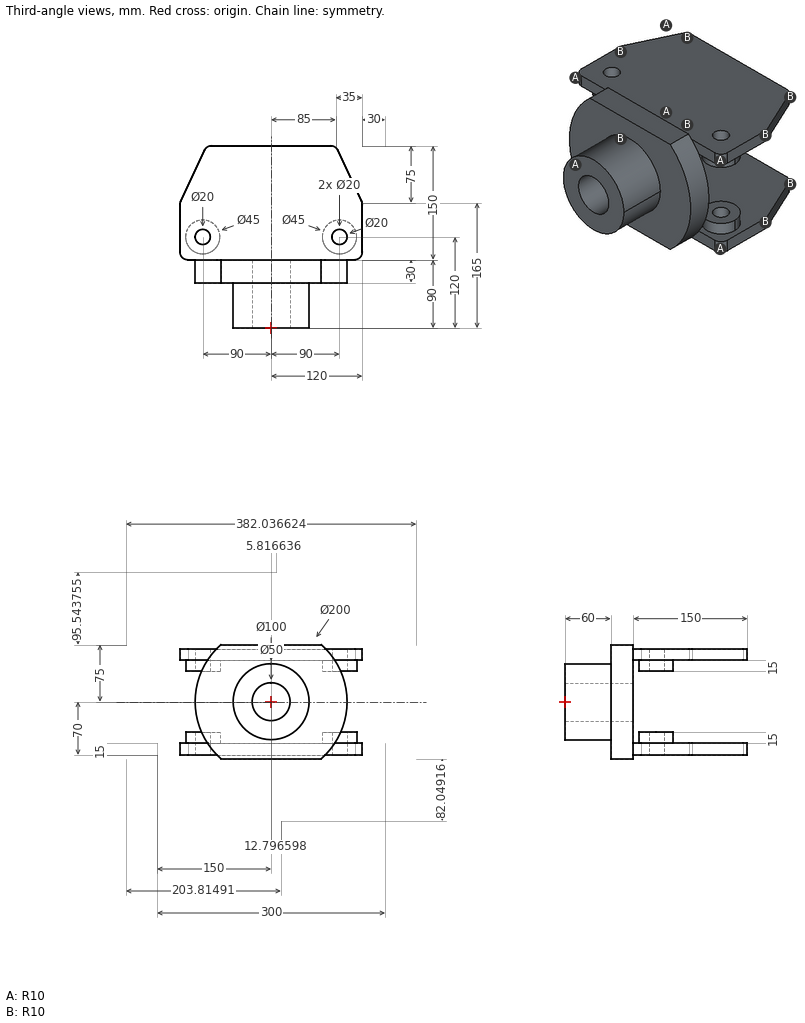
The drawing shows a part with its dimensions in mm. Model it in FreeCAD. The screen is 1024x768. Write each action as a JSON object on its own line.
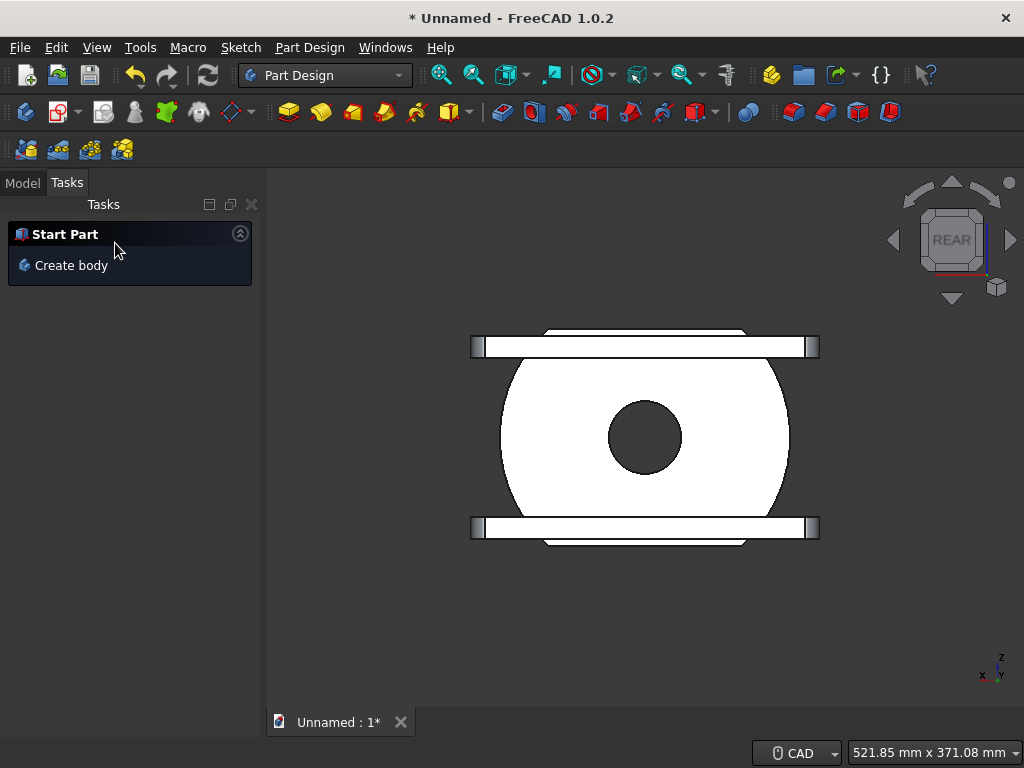
{"action": "key", "text": "5"}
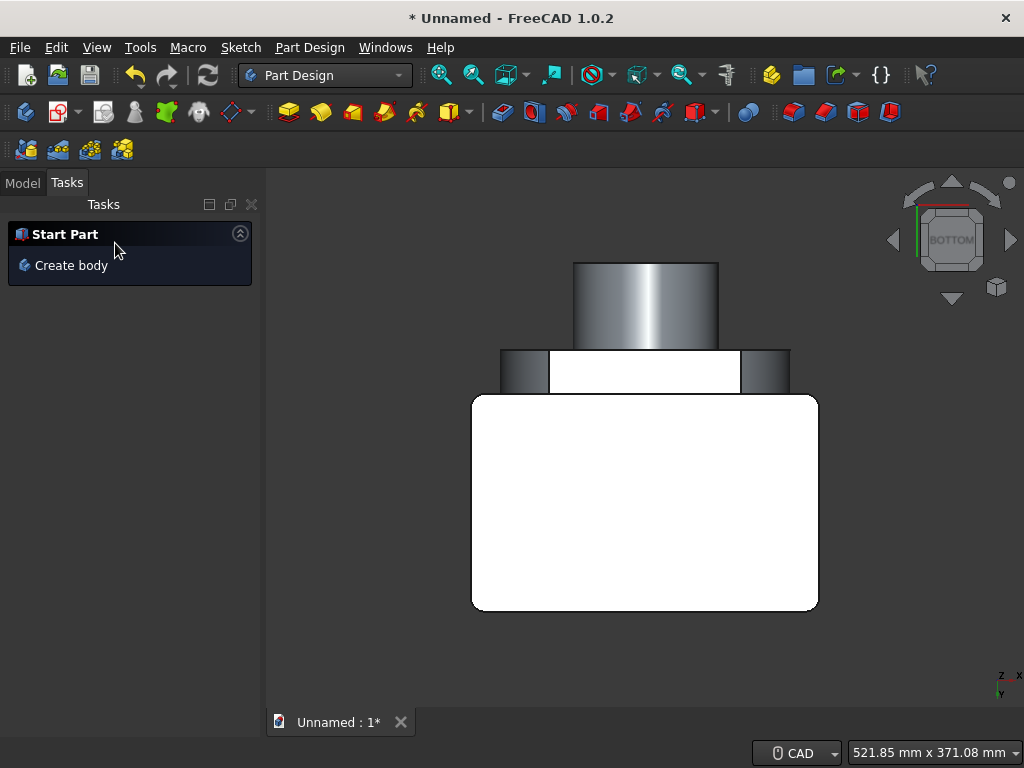
{"action": "left_click", "coordinate": [695, 502]}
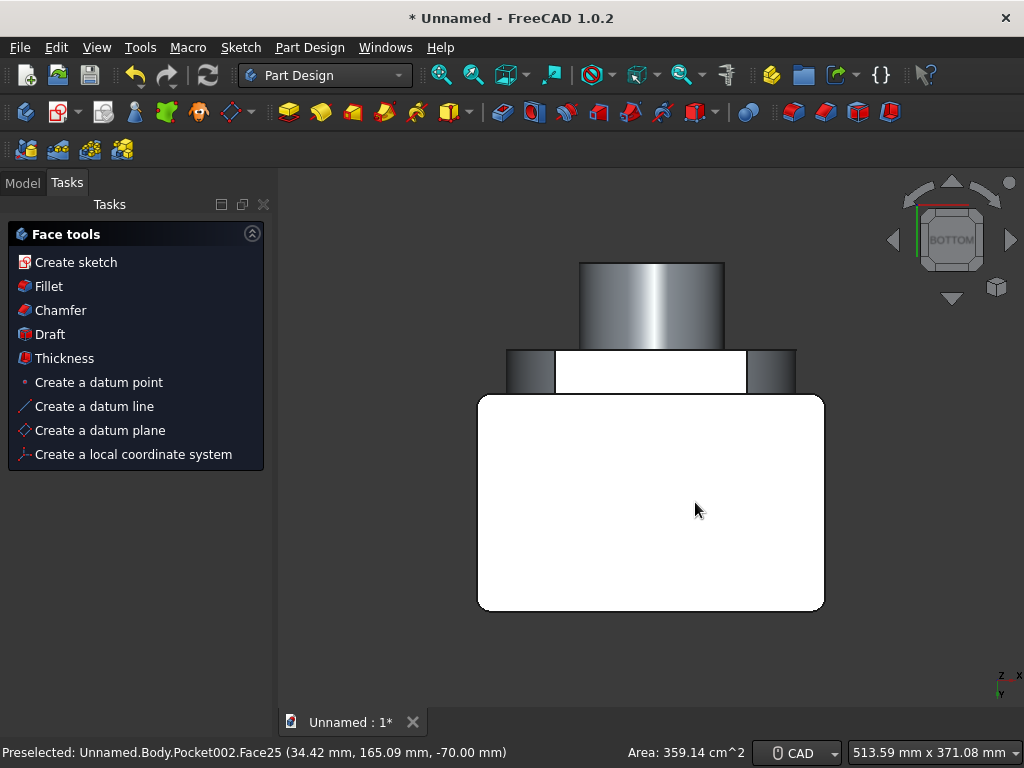
{"action": "left_click", "coordinate": [58, 112]}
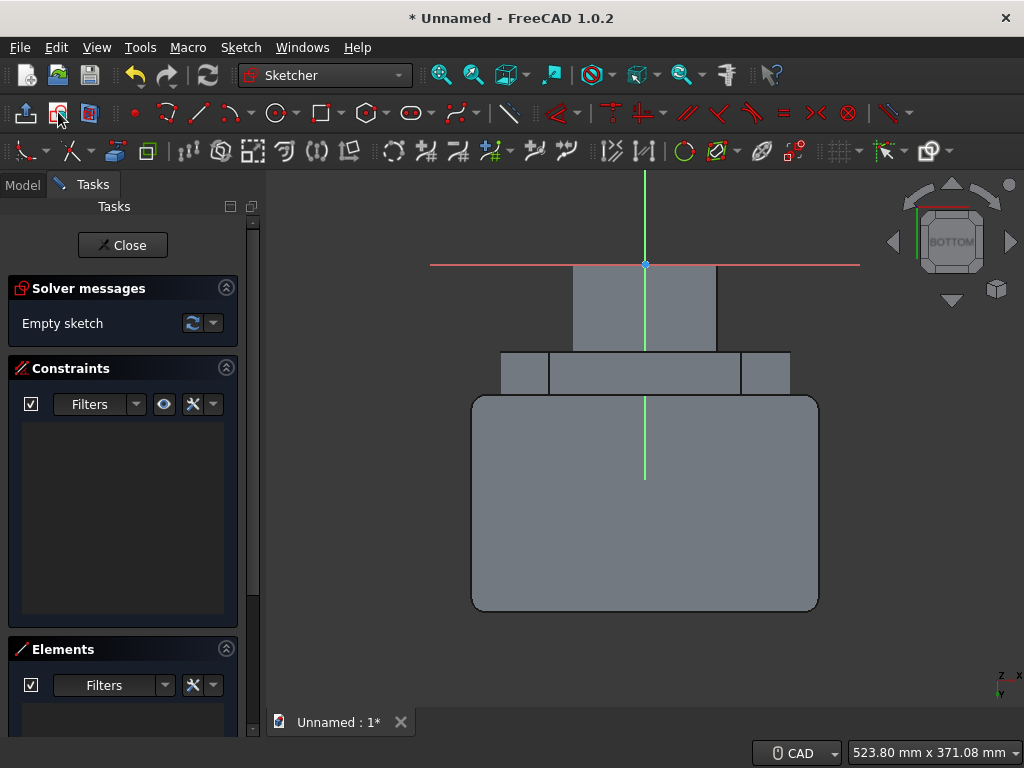
{"action": "left_click", "coordinate": [90, 114]}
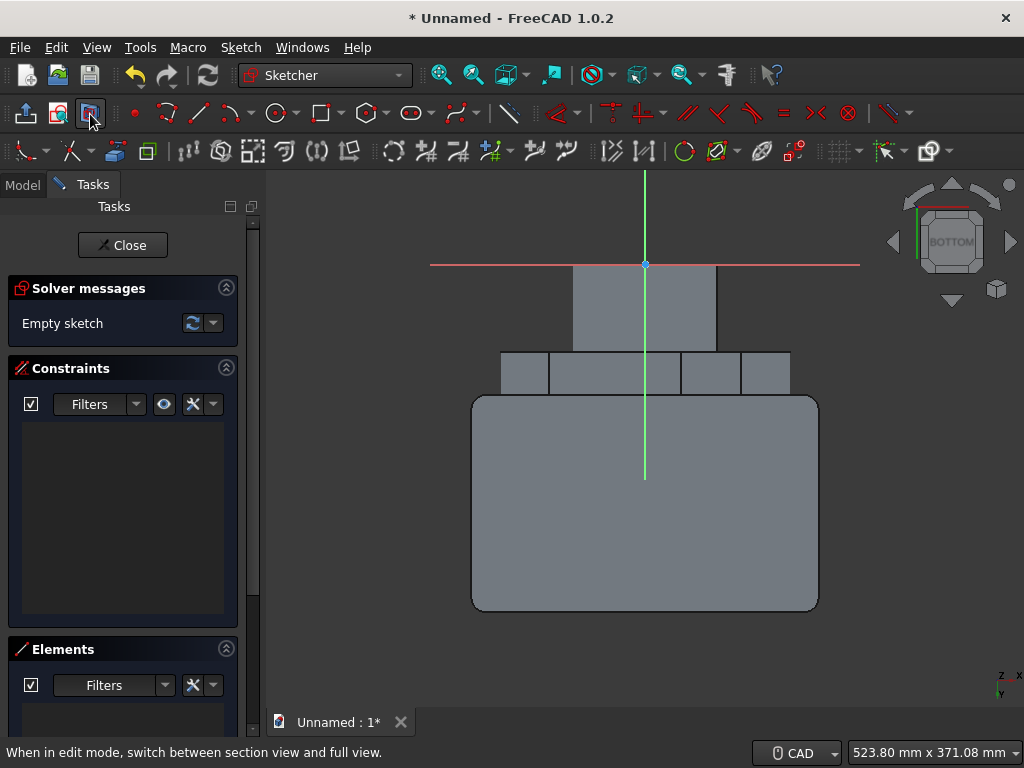
{"action": "scroll", "coordinate": [784, 198], "scroll_direction": "up", "scroll_amount": 2}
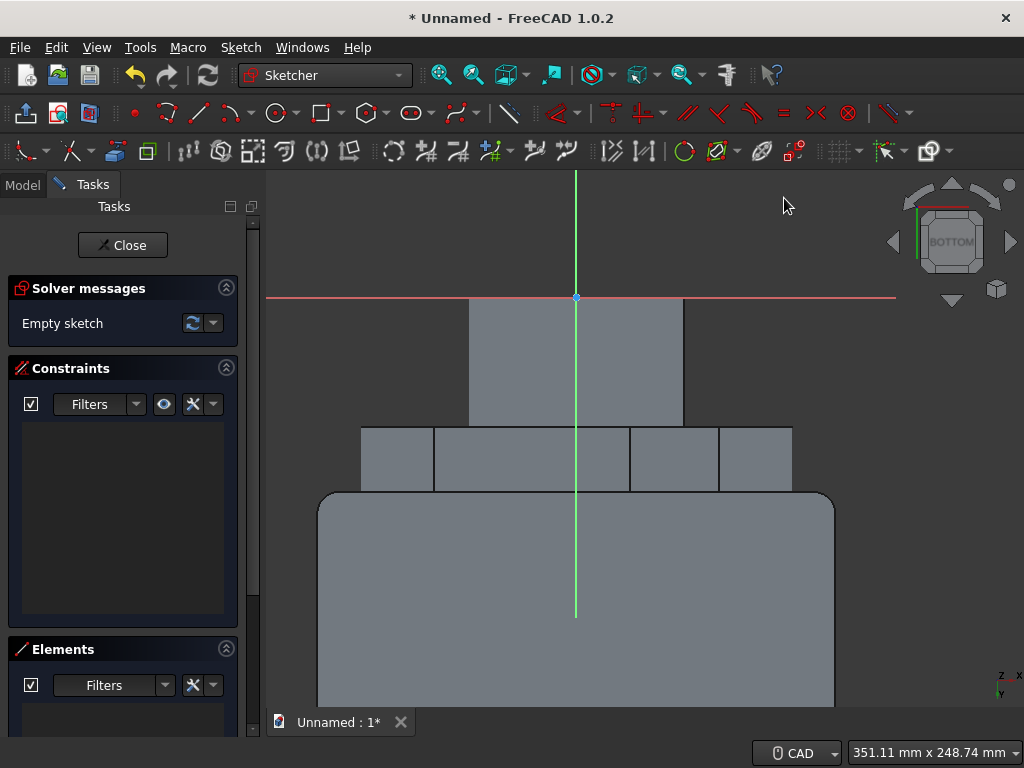
{"action": "left_click", "coordinate": [276, 114]}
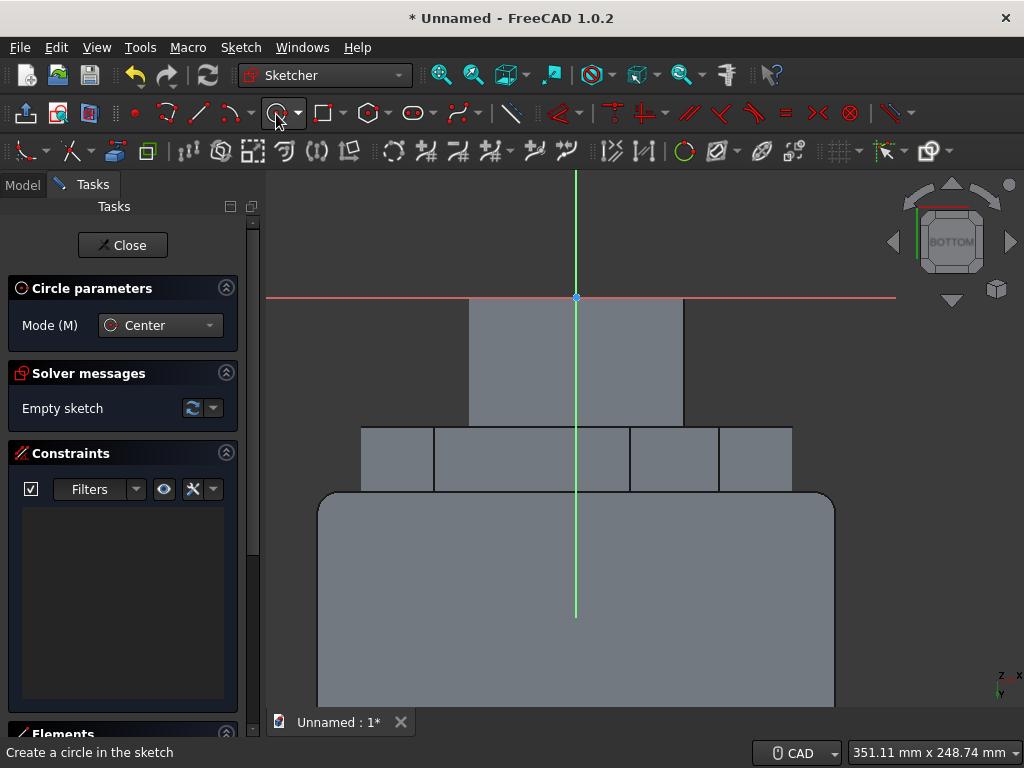
{"action": "left_click", "coordinate": [771, 557]}
{"action": "left_click", "coordinate": [786, 541]}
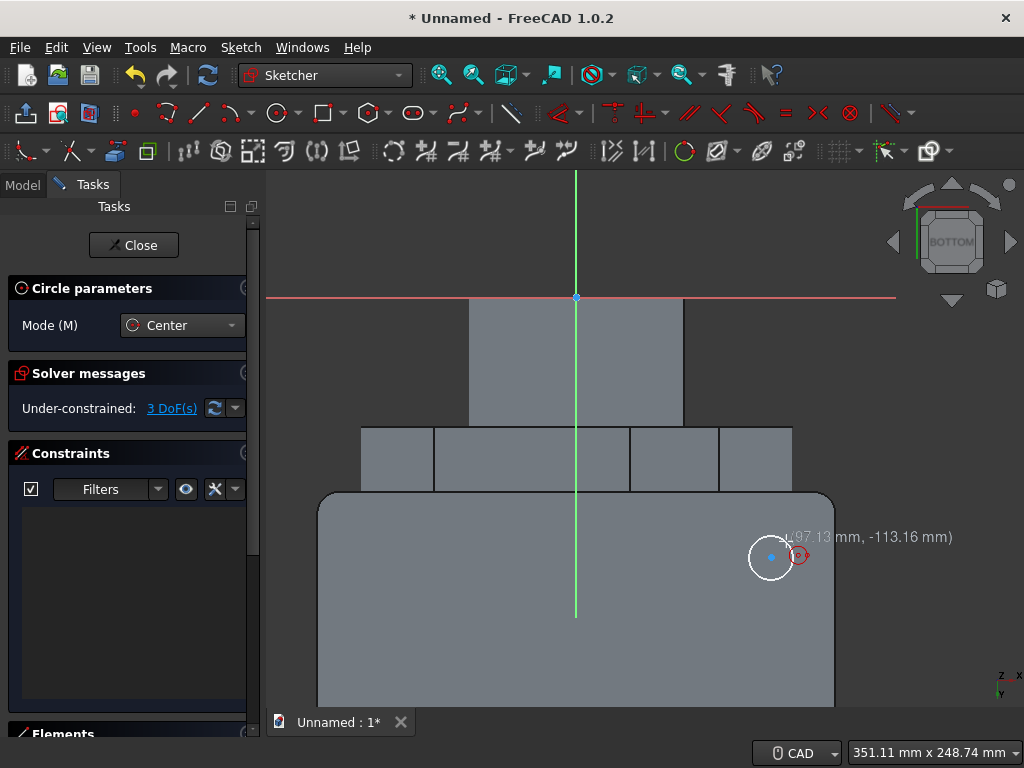
{"action": "left_click", "coordinate": [382, 557]}
{"action": "left_click", "coordinate": [397, 541]}
{"action": "key", "text": "Escape"}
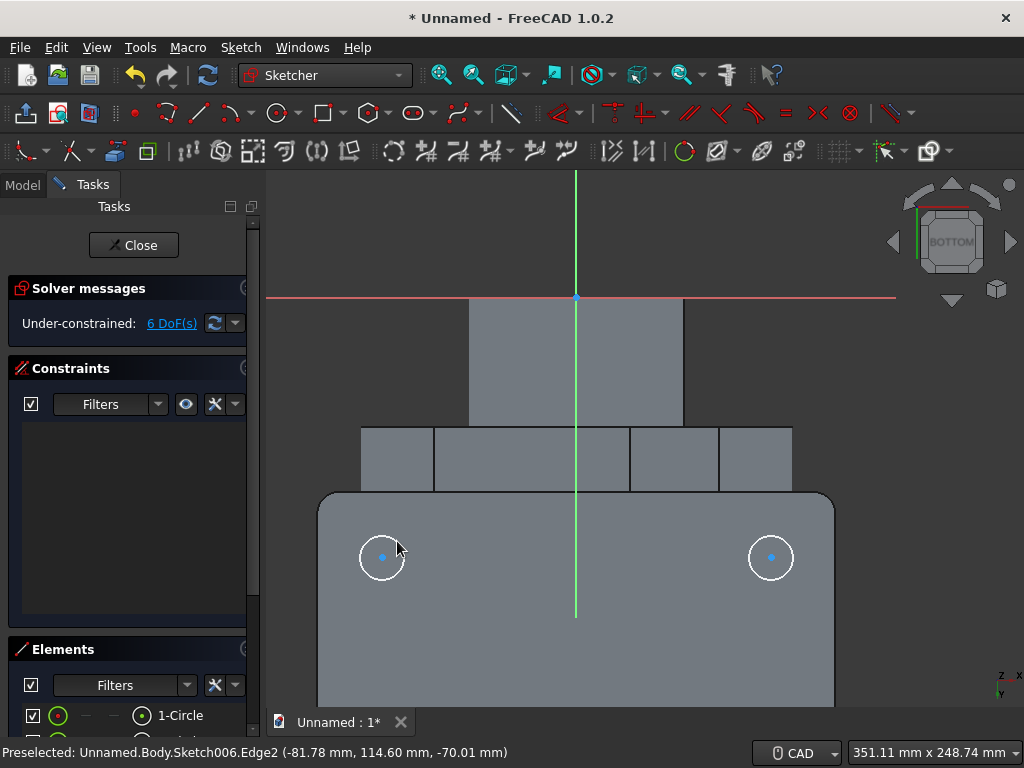
{"action": "left_click", "coordinate": [786, 542]}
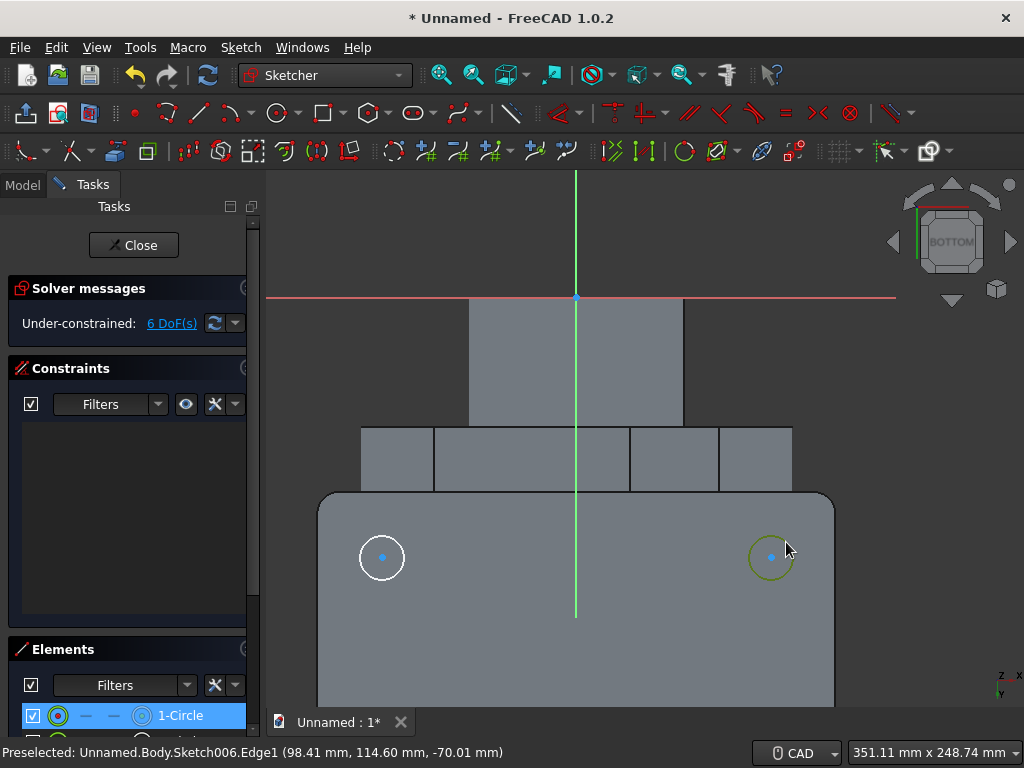
{"action": "left_click", "coordinate": [397, 542]}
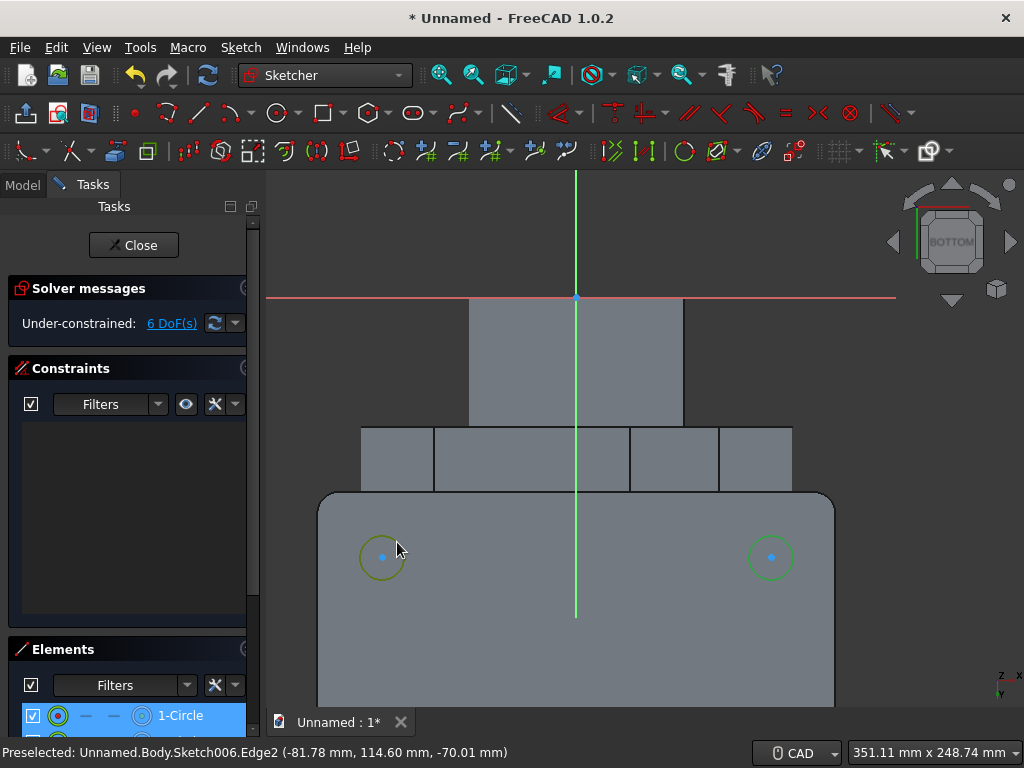
{"action": "key", "text": "e"}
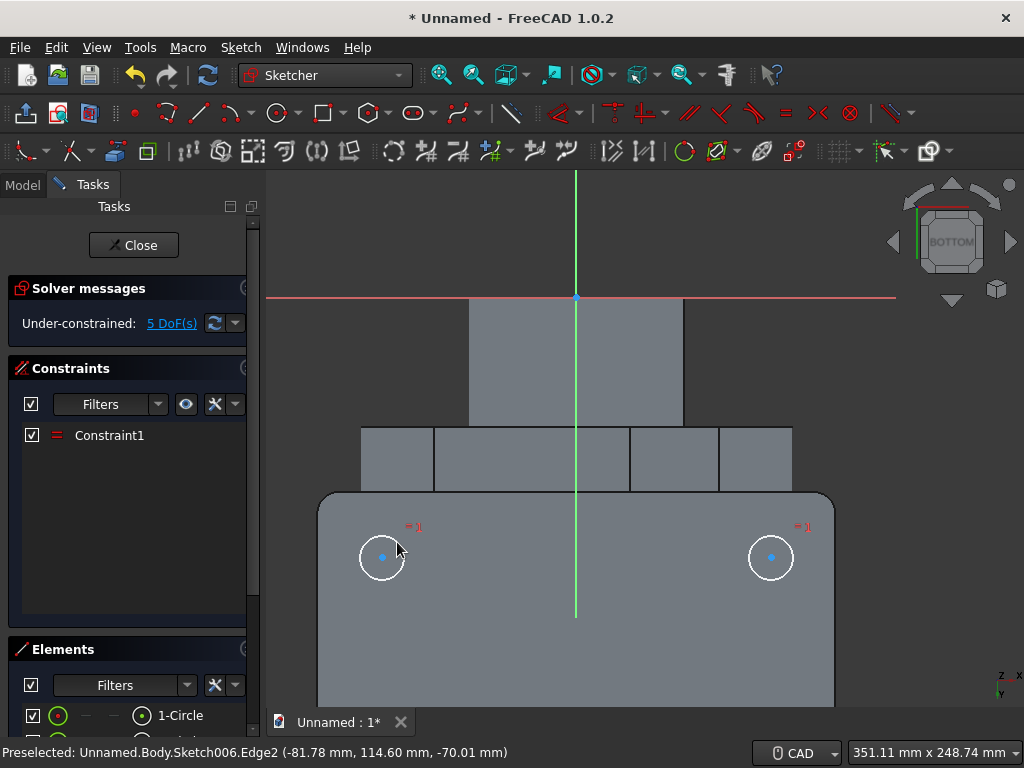
{"action": "left_click", "coordinate": [771, 558]}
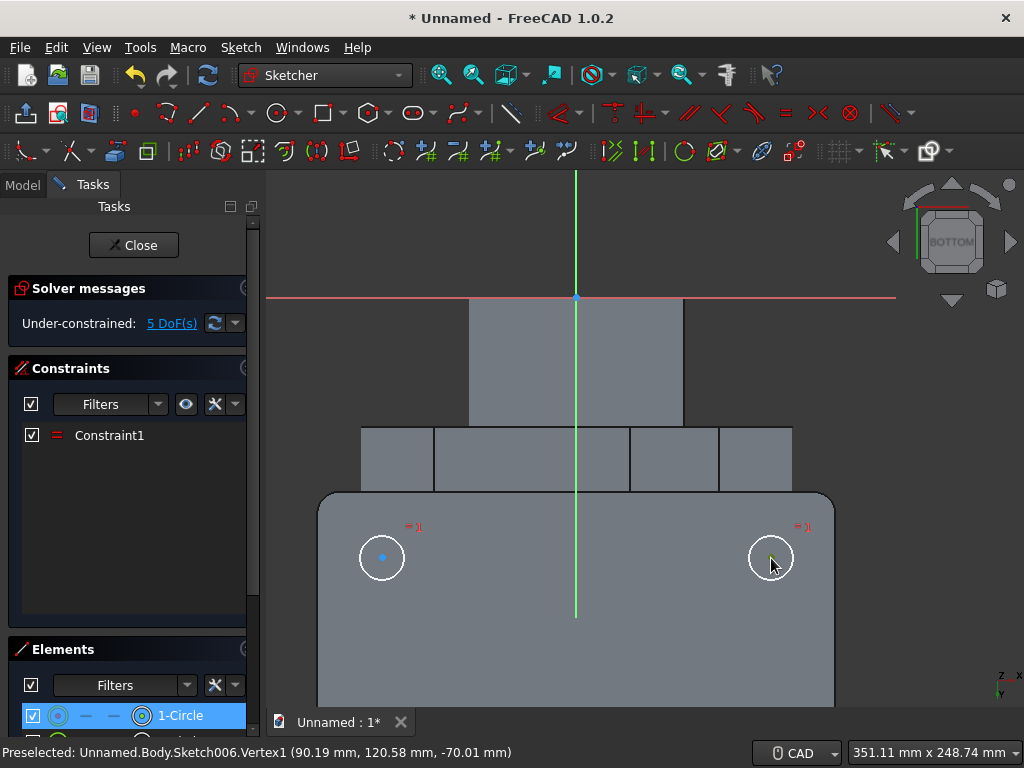
{"action": "left_click", "coordinate": [382, 558]}